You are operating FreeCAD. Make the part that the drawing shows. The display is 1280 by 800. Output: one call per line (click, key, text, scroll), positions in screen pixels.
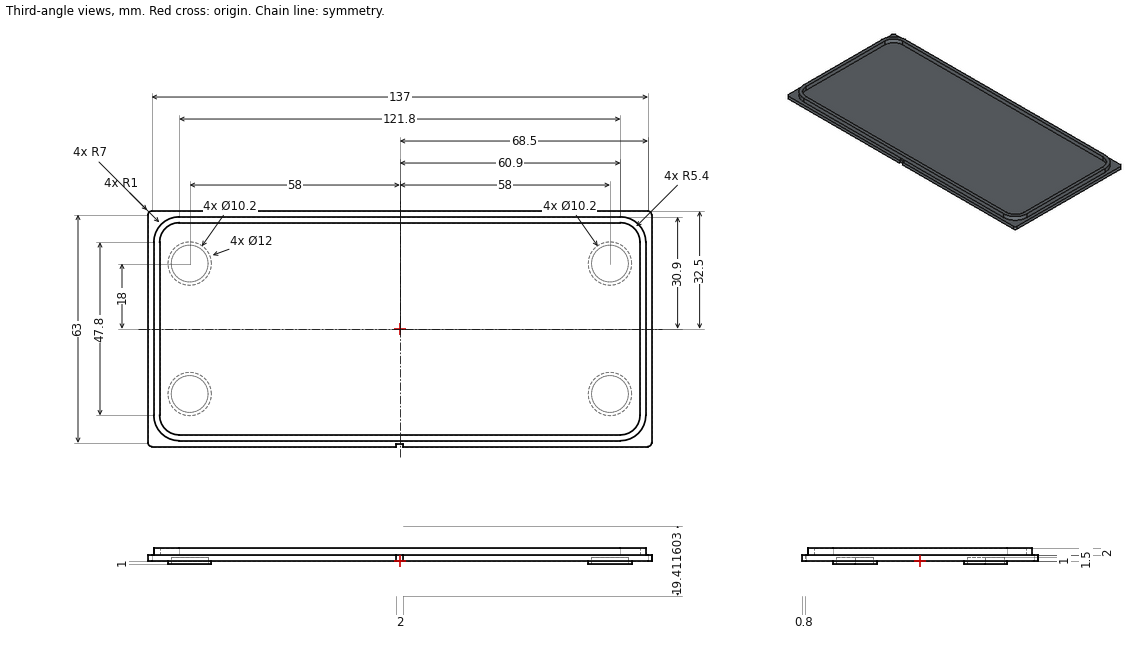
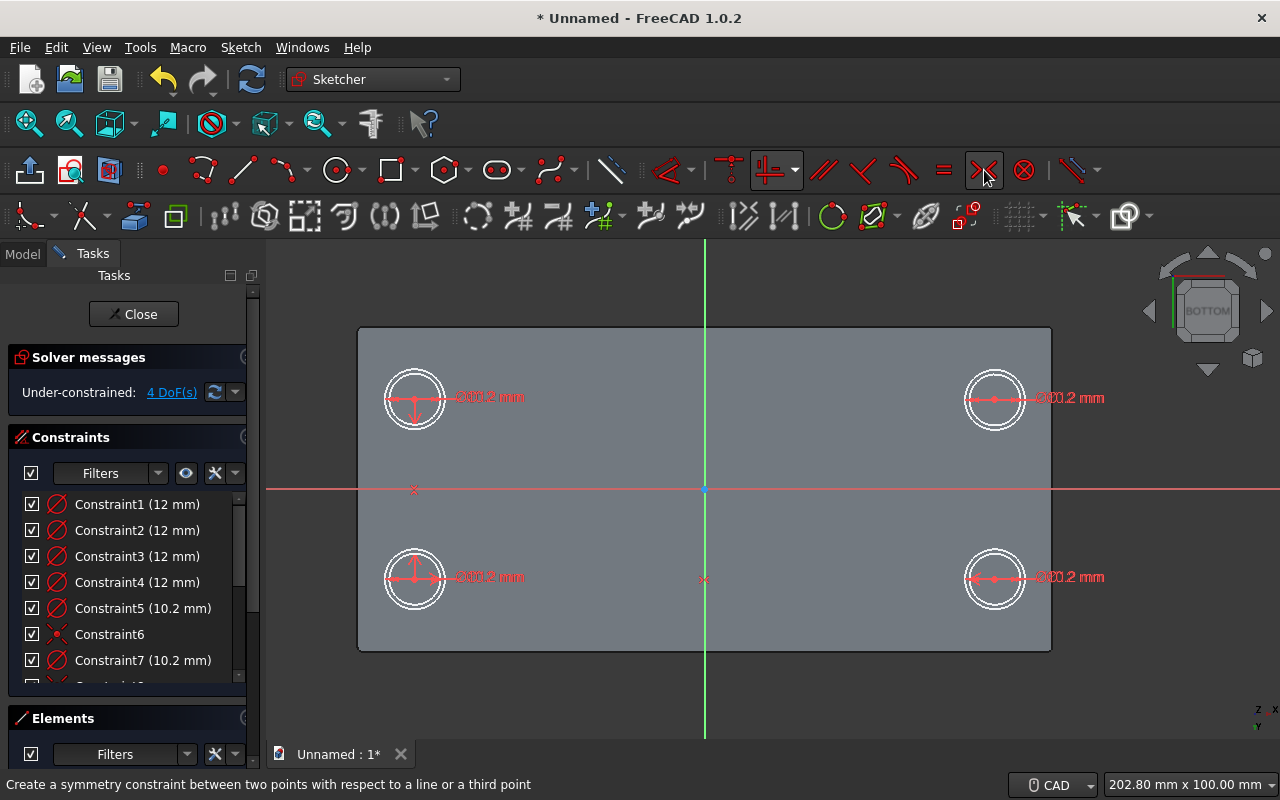
click(995, 579)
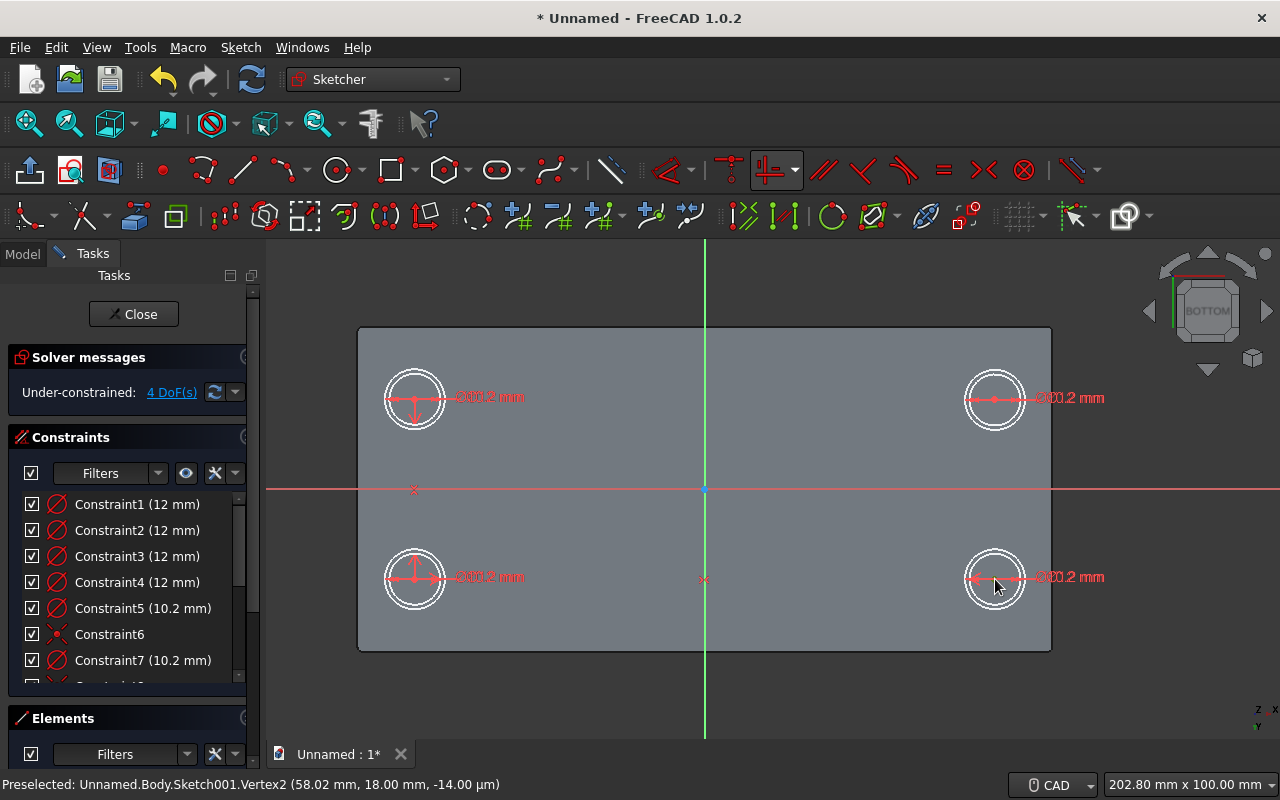
click(995, 400)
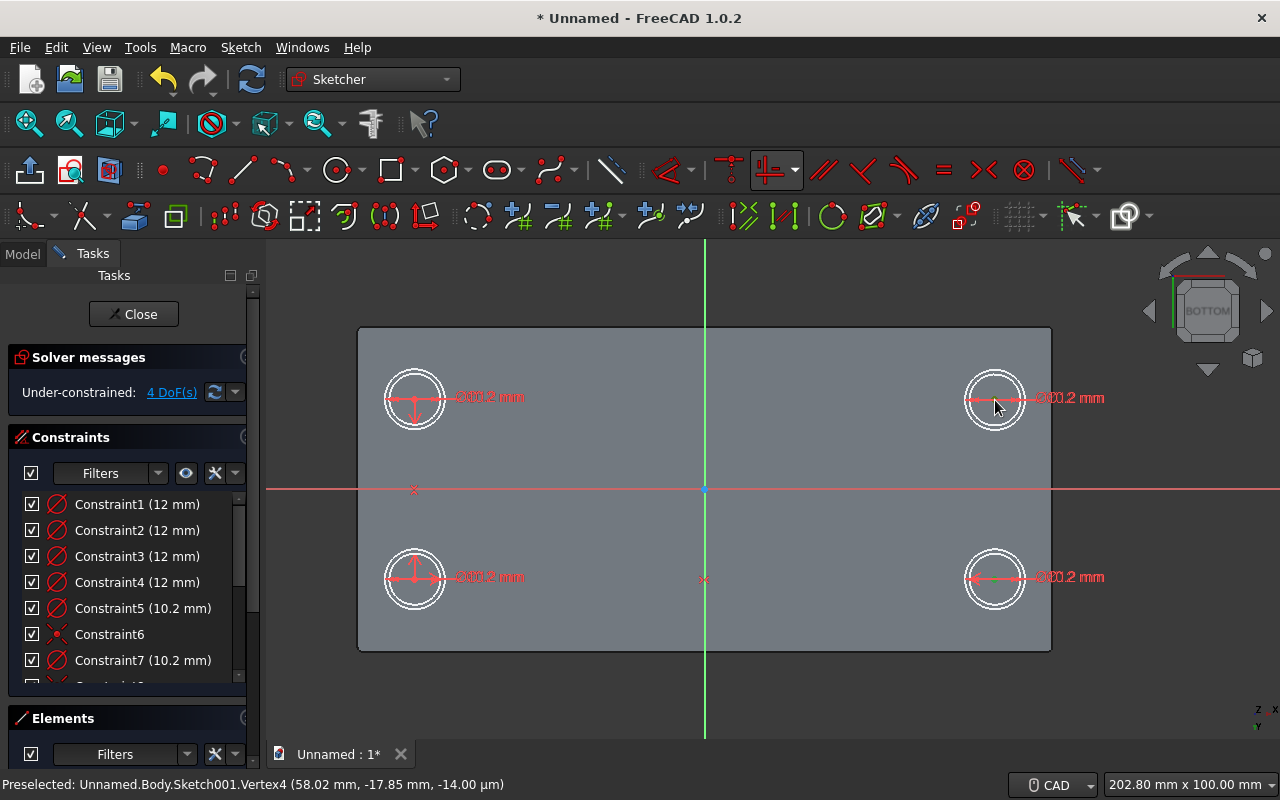
click(353, 489)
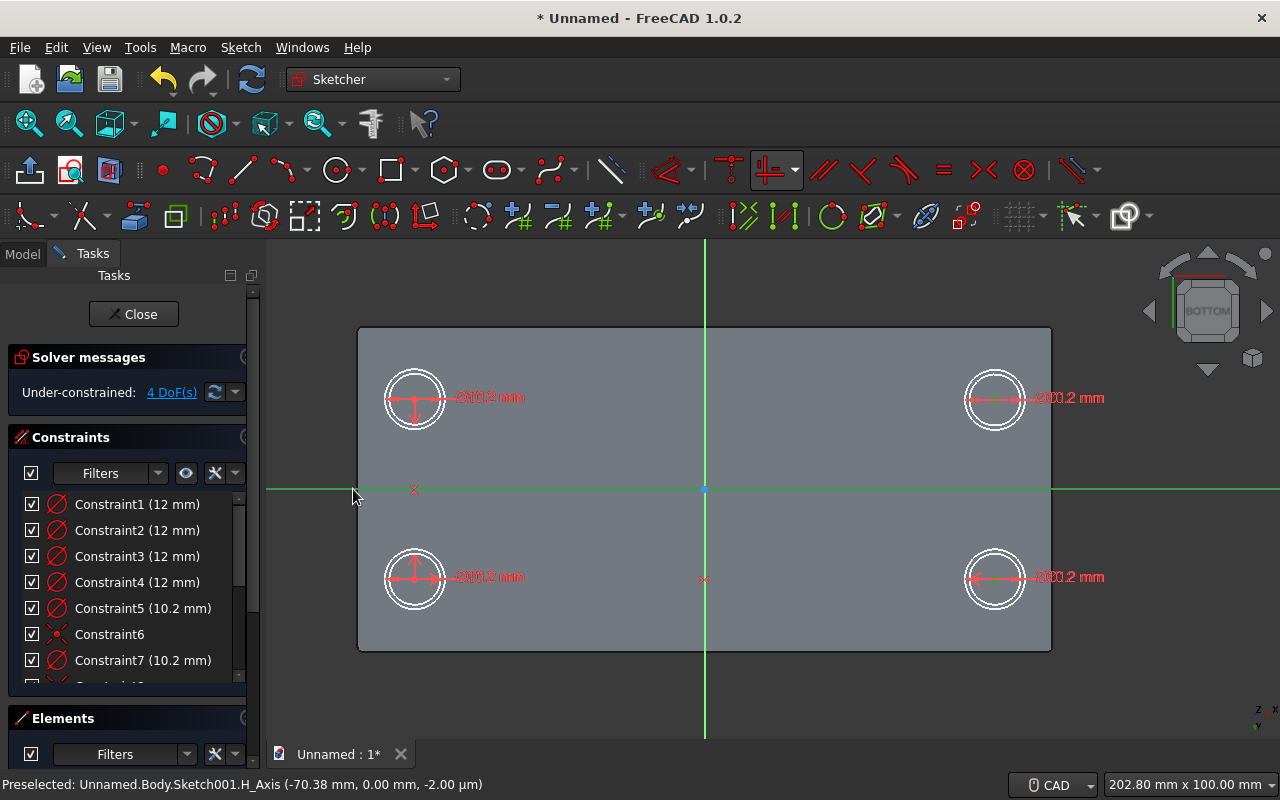
click(984, 170)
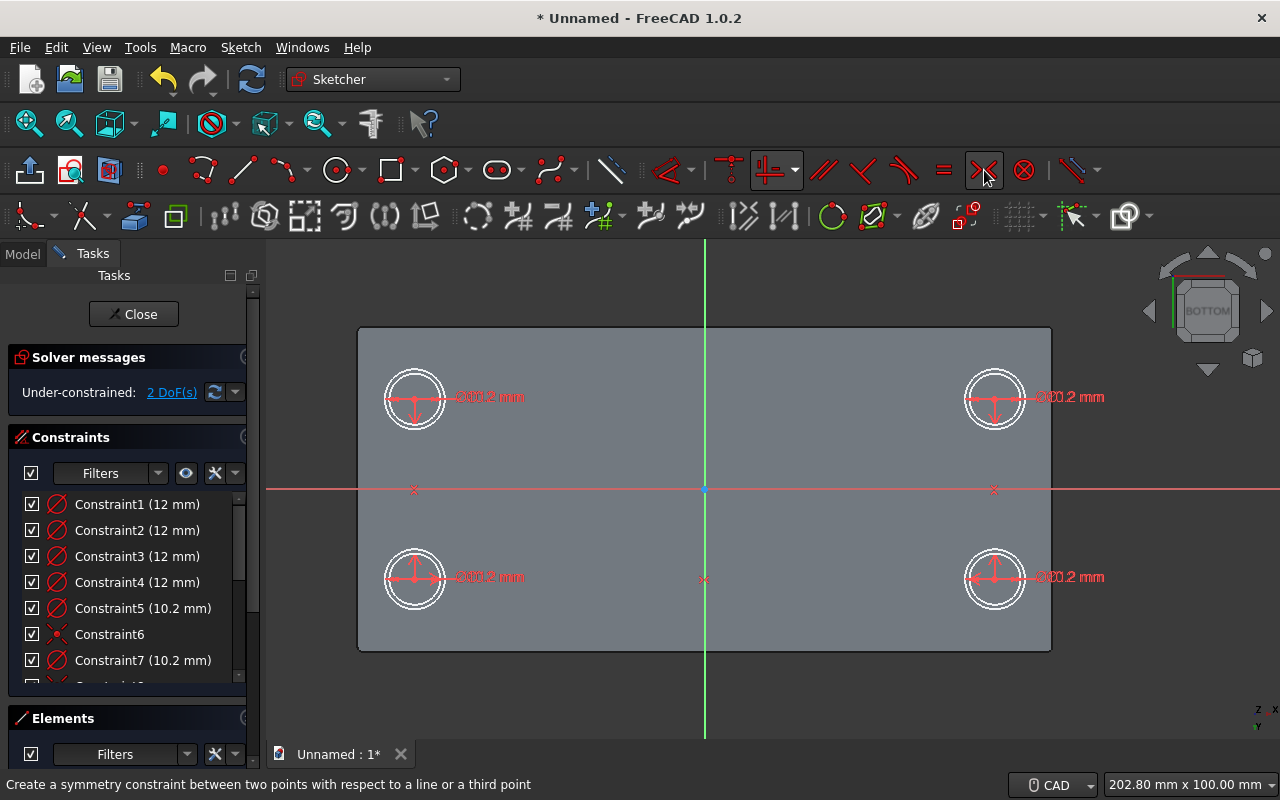
click(666, 170)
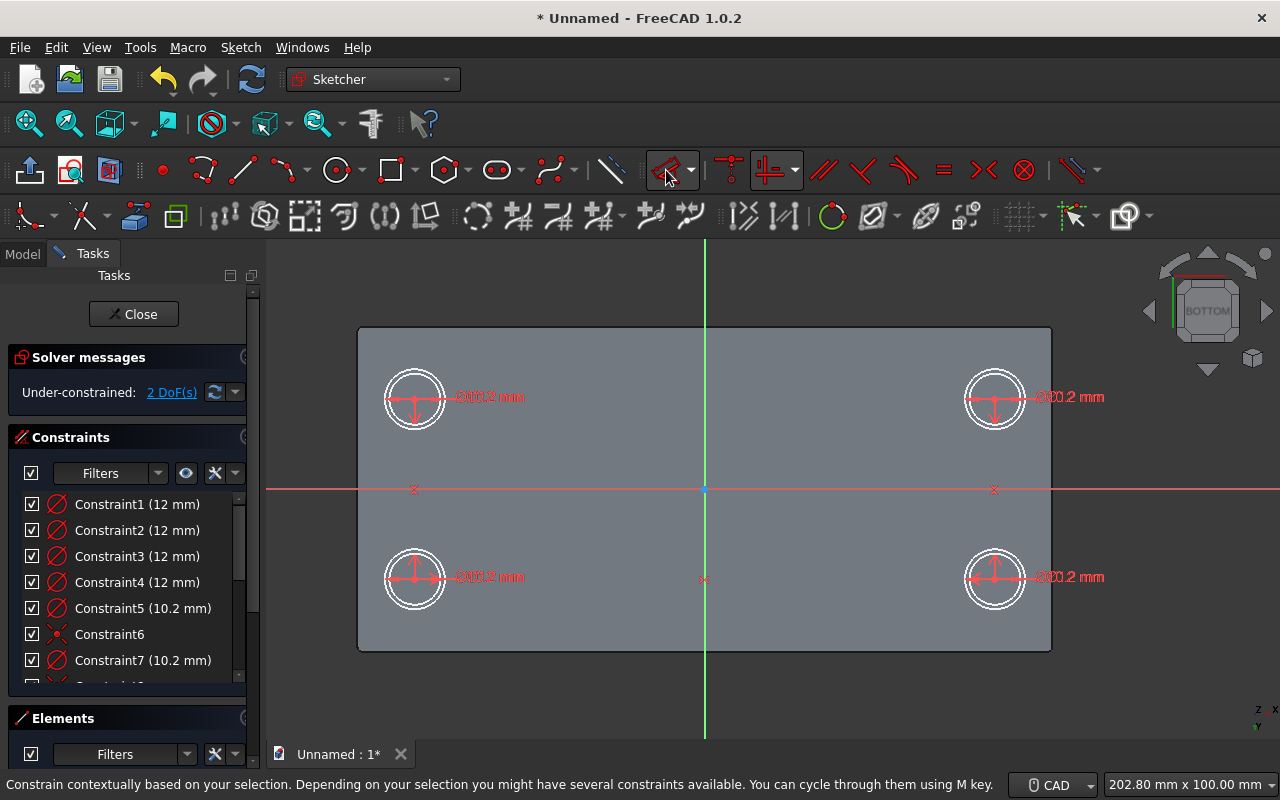
click(415, 579)
click(560, 613)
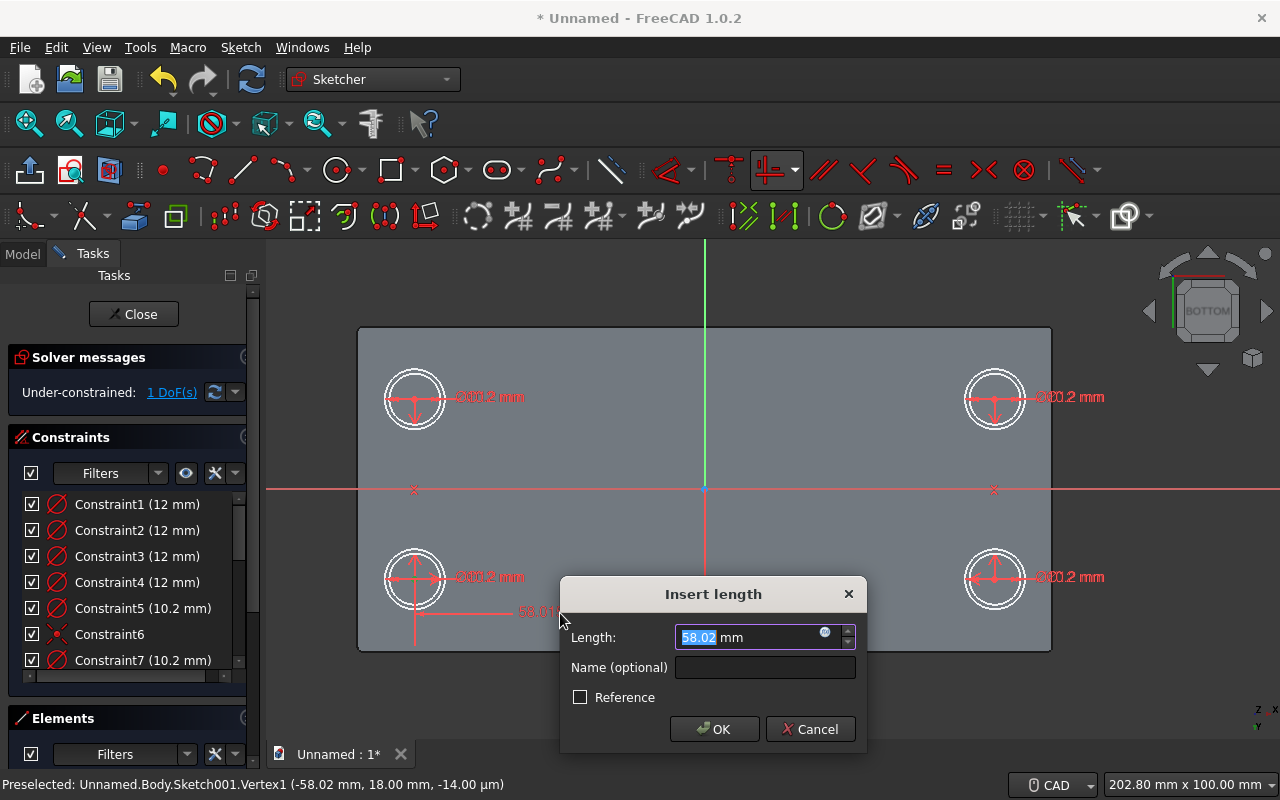
text(58)
key(Return)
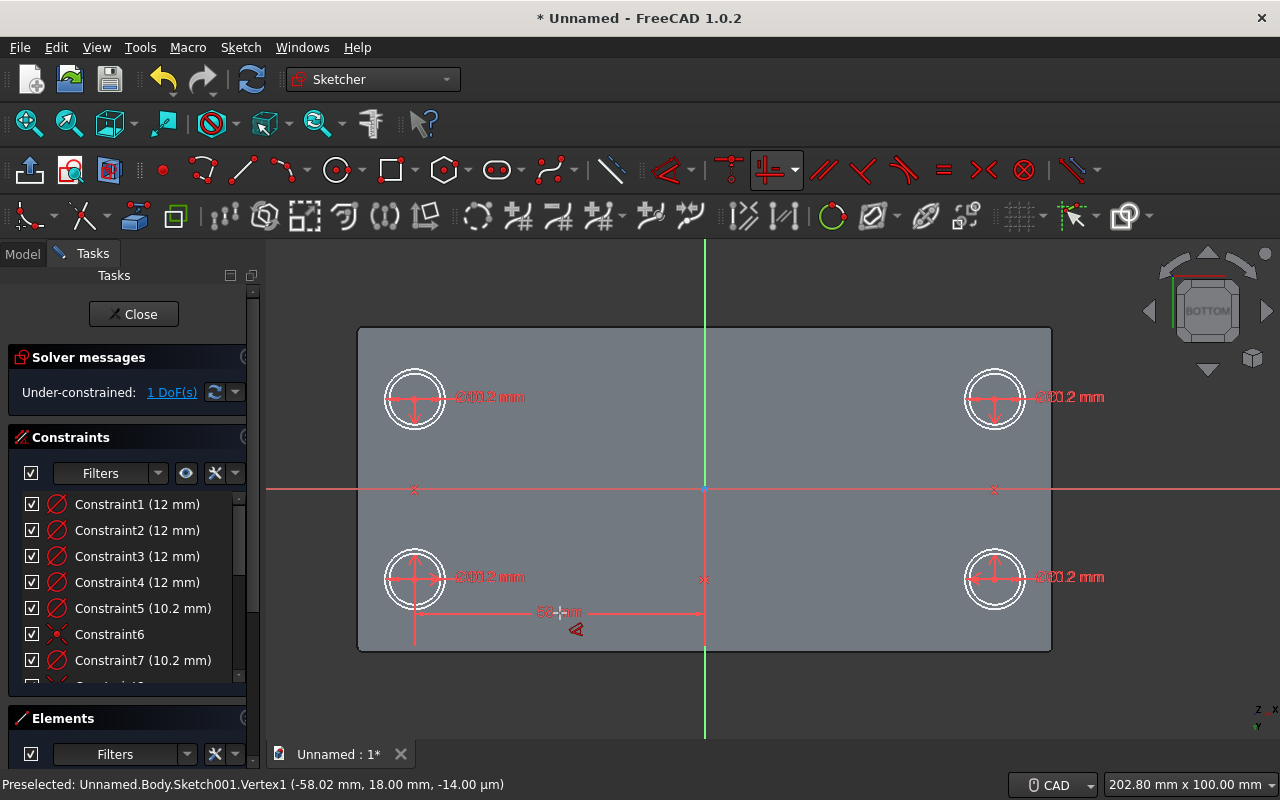
click(415, 579)
click(381, 534)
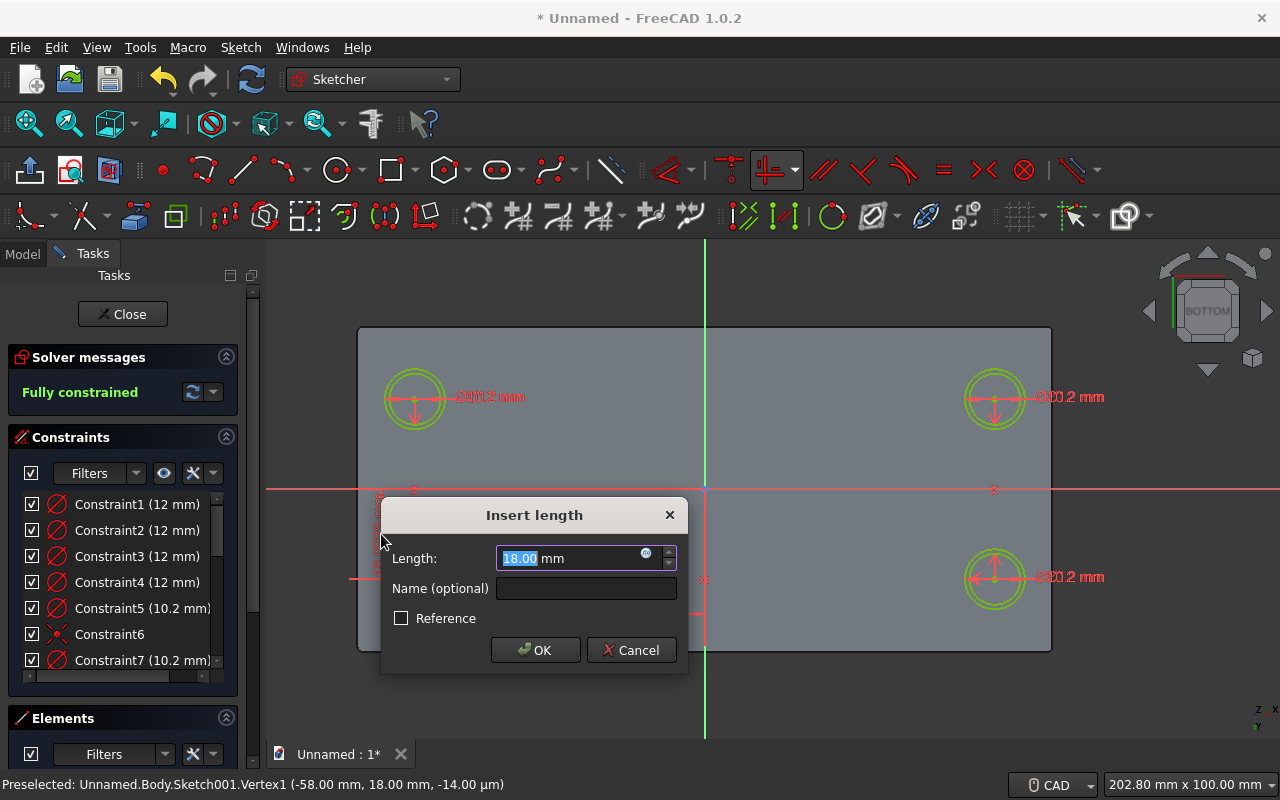
text(18)
key(Return)
key(Escape)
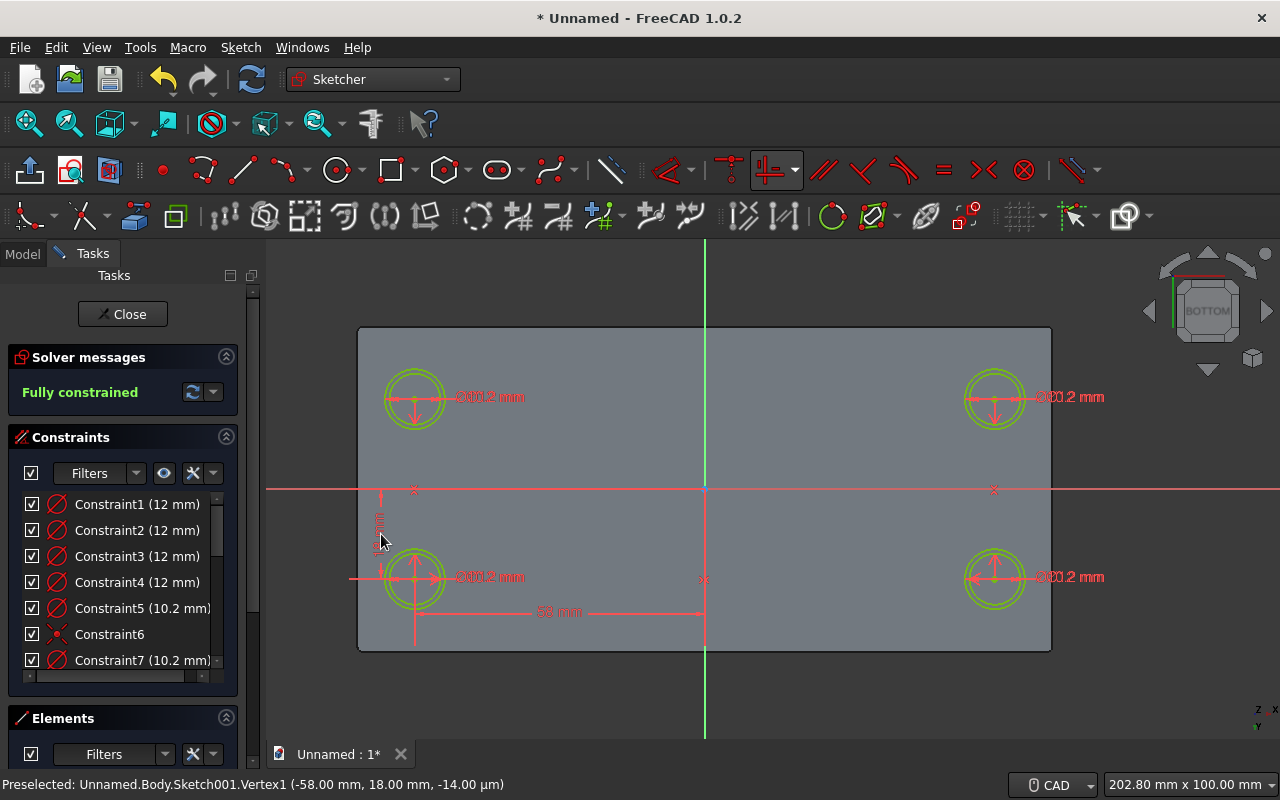
click(123, 314)